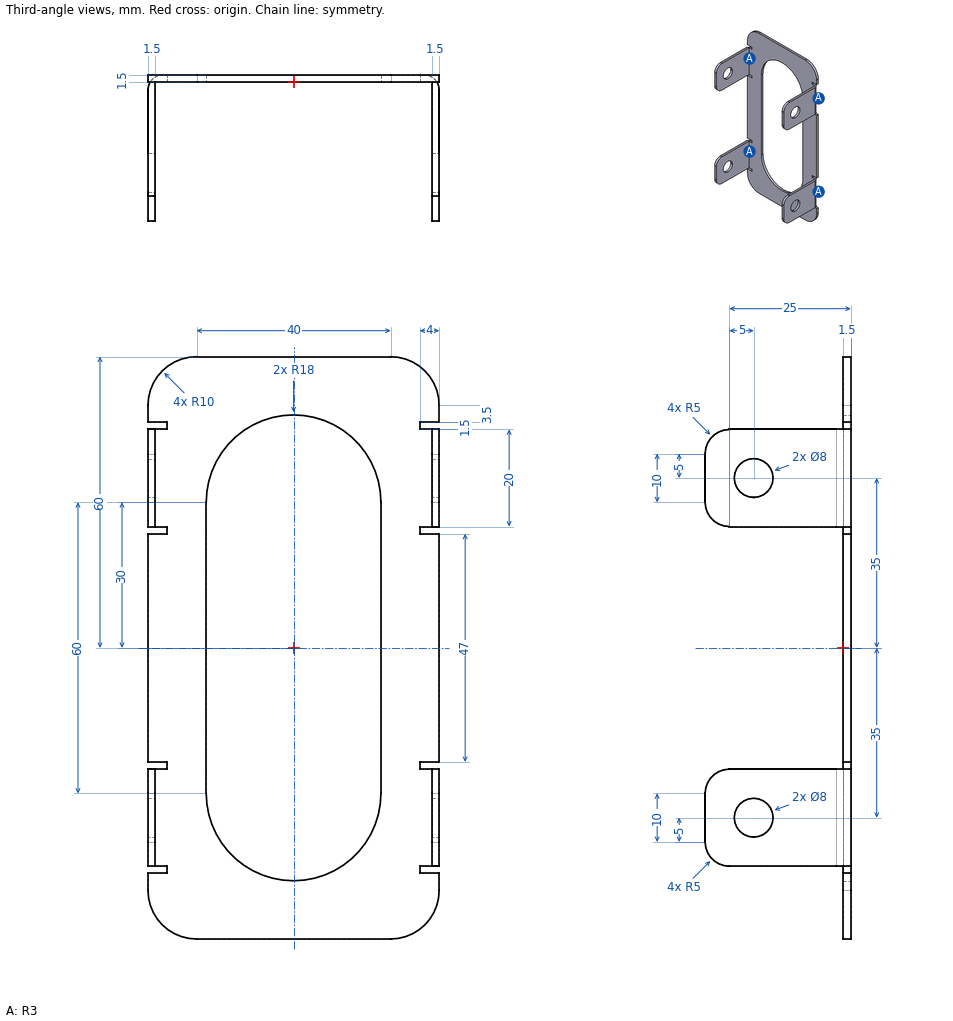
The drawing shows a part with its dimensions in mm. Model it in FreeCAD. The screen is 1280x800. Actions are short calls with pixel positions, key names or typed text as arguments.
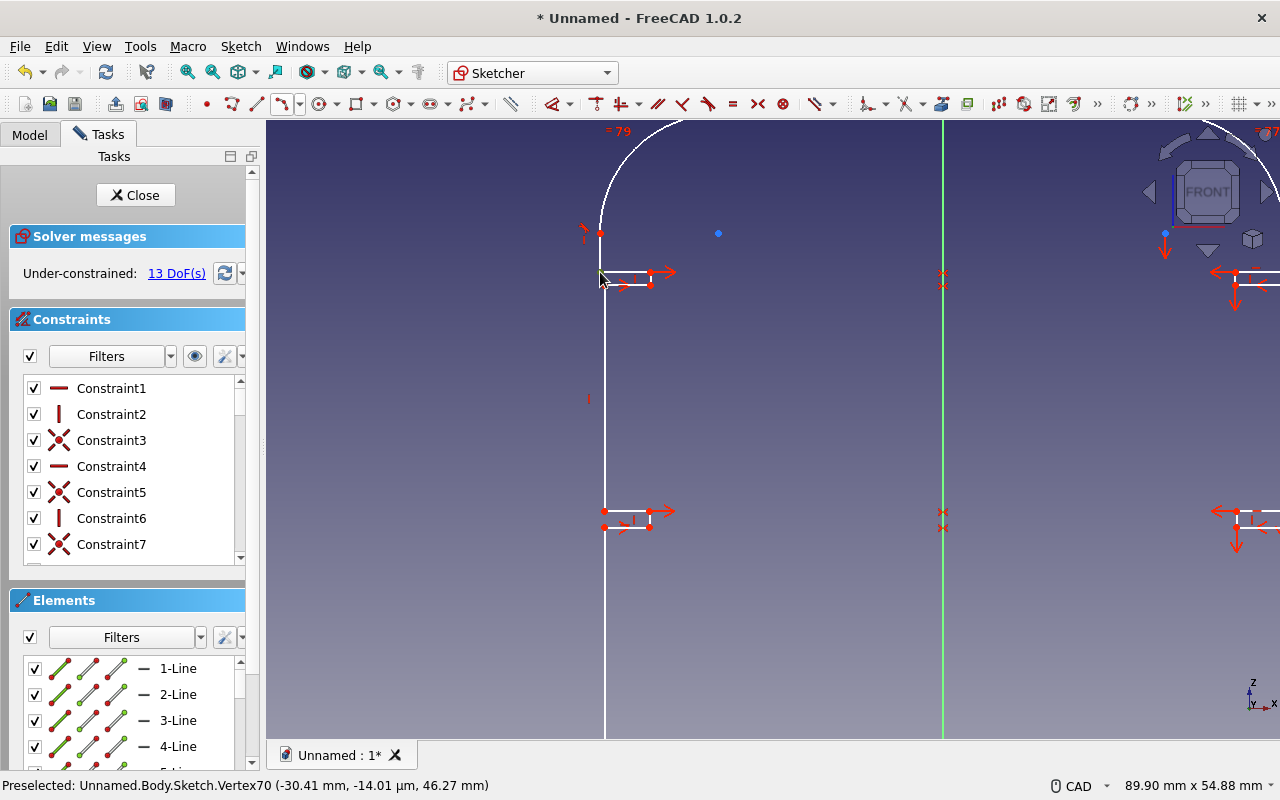
scroll(602, 272, down, 6)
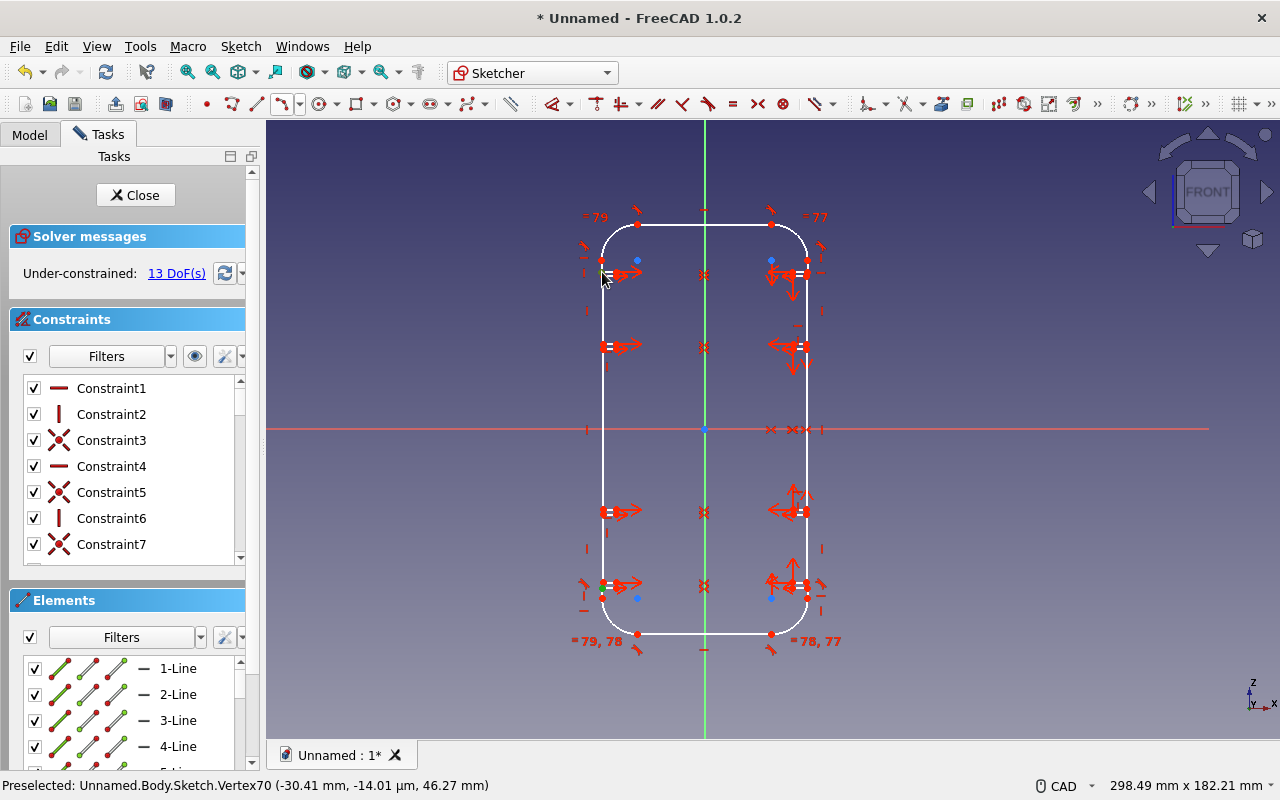
click(353, 429)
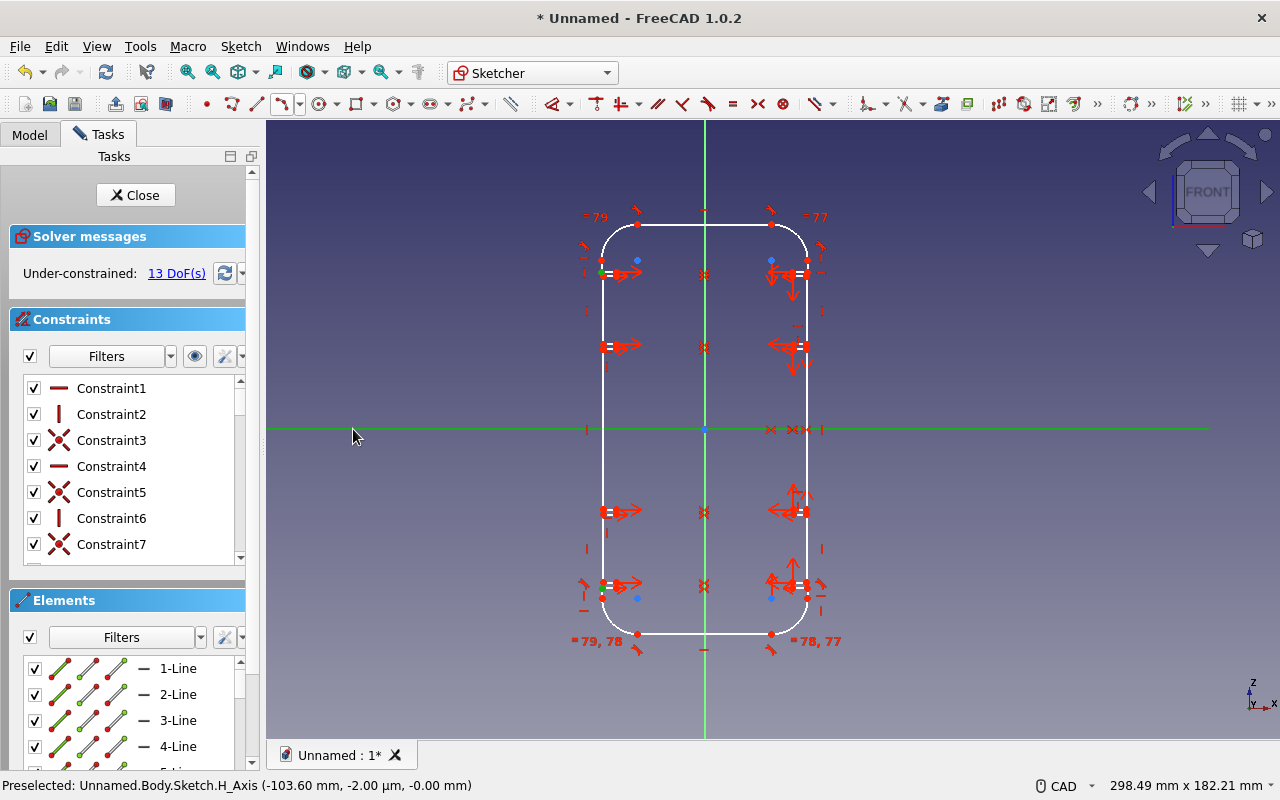
click(758, 104)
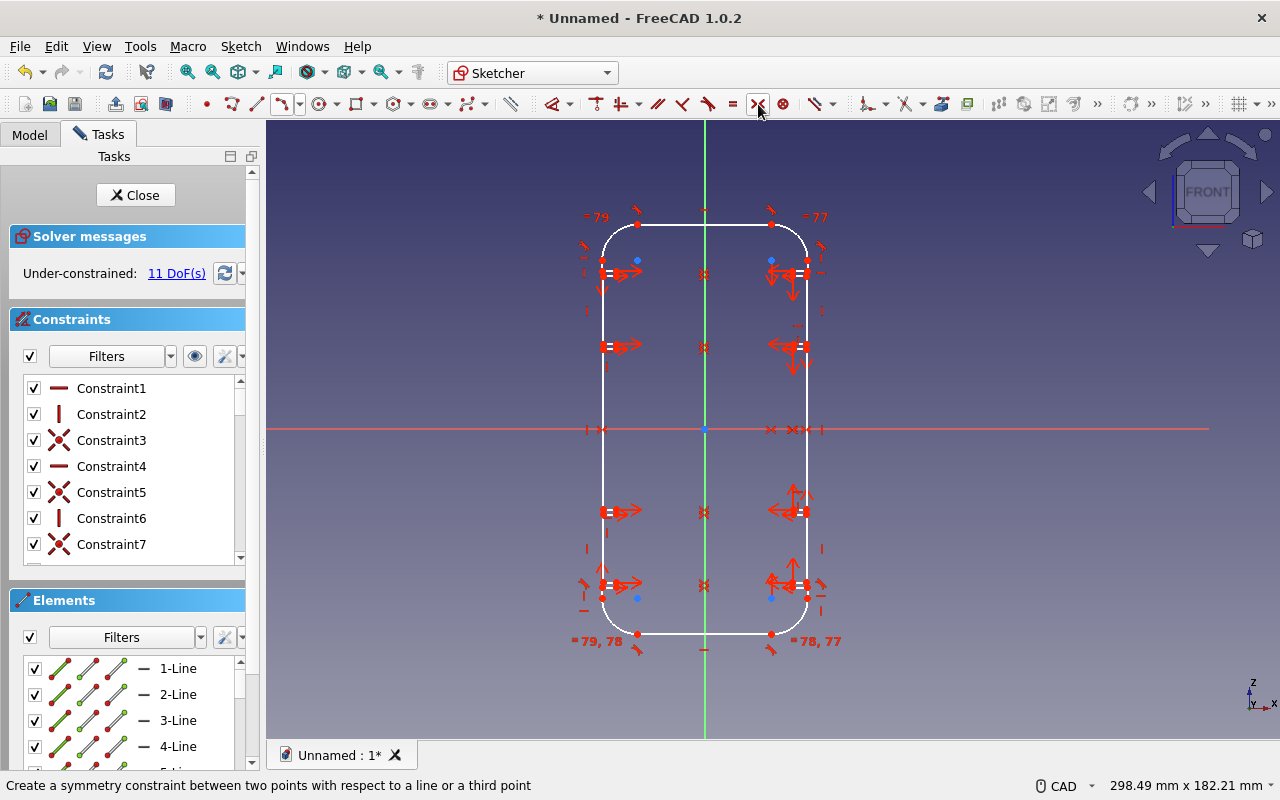
click(804, 244)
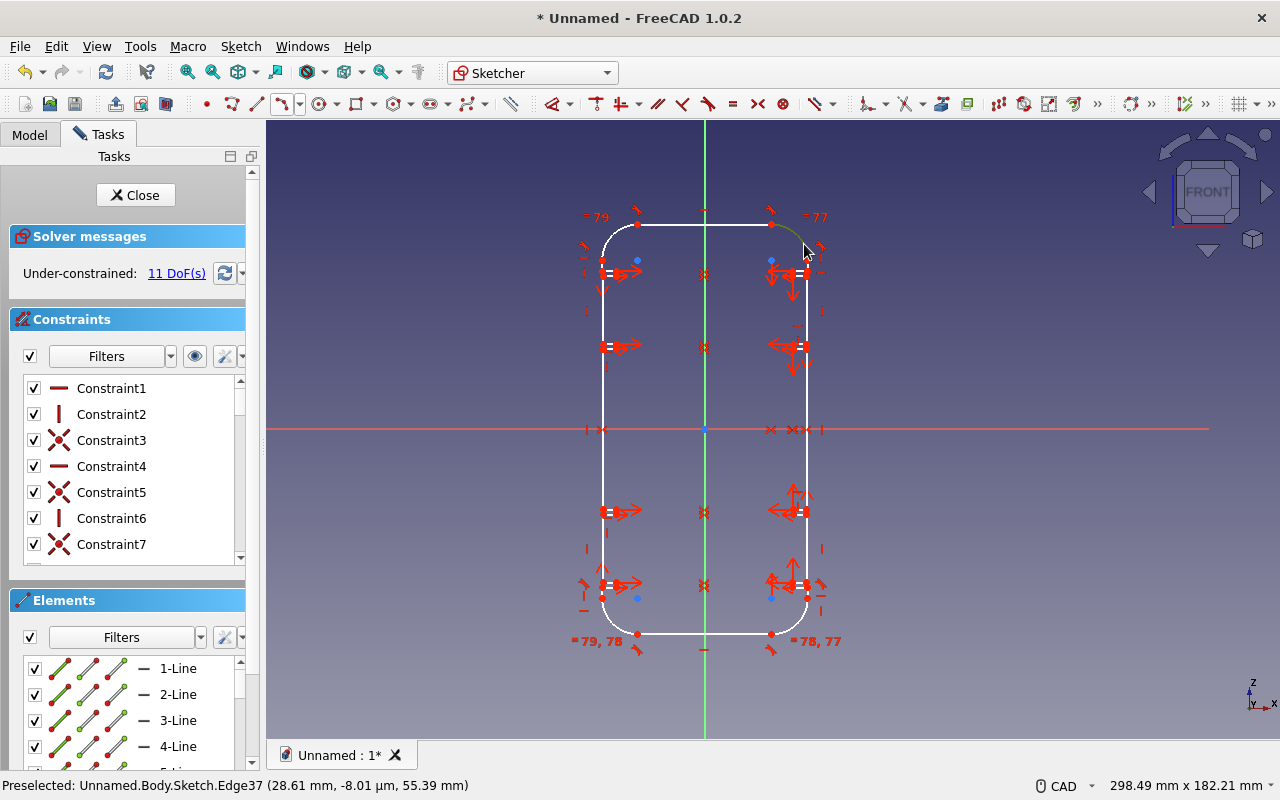
key(k)
key(r)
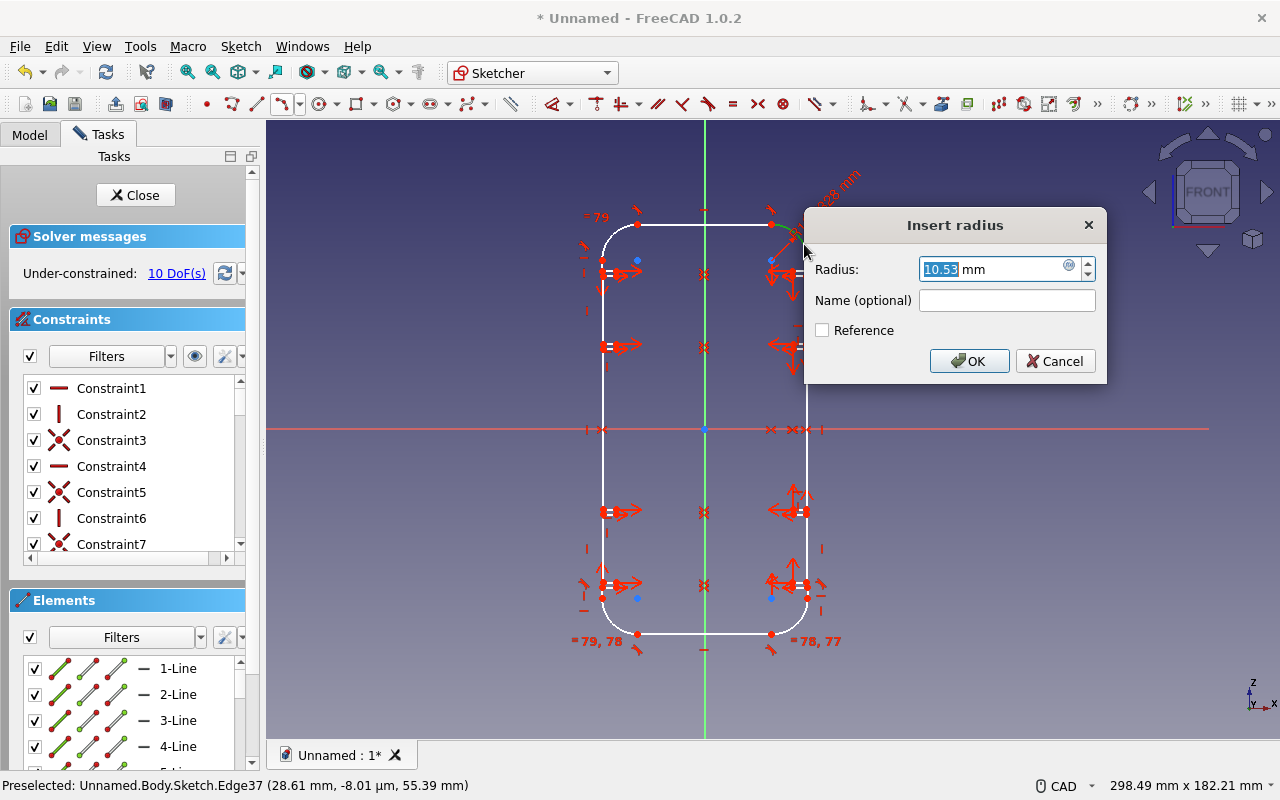
text(10)
key(Return)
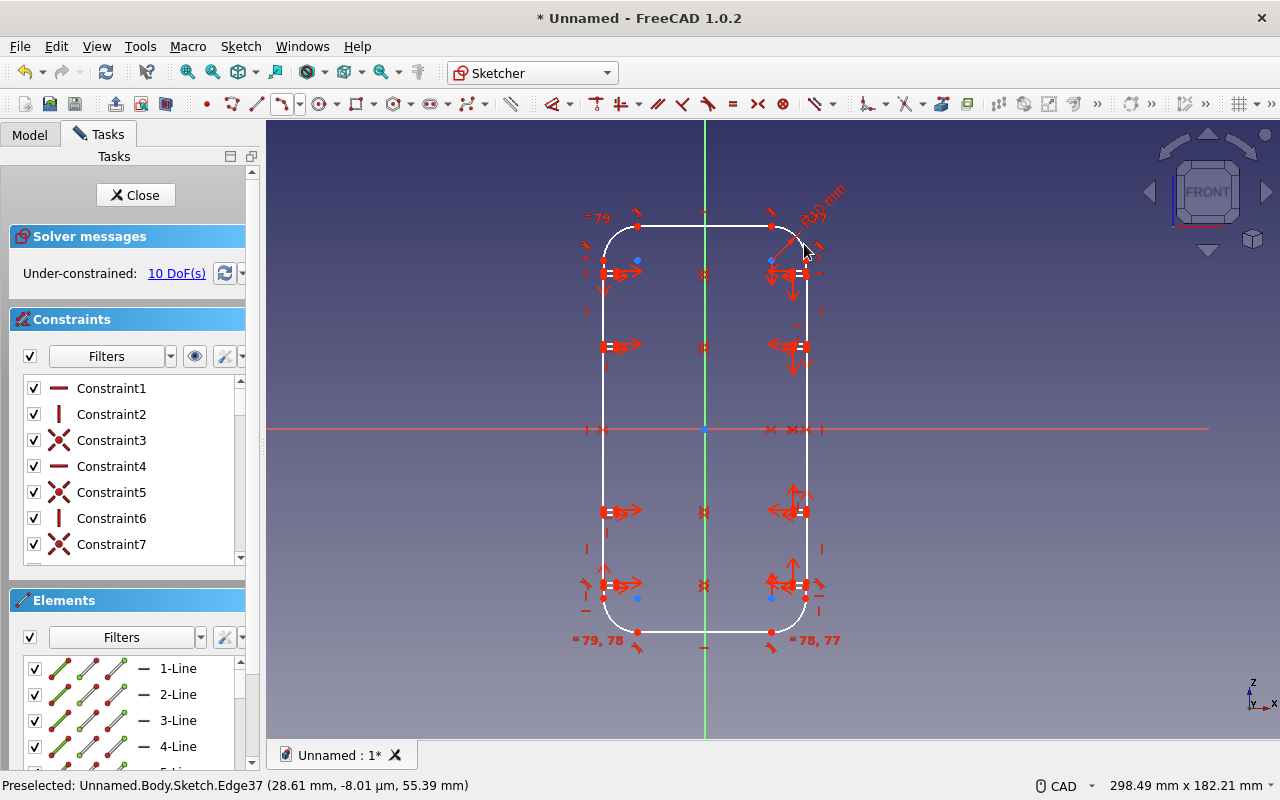
scroll(801, 271, up, 6)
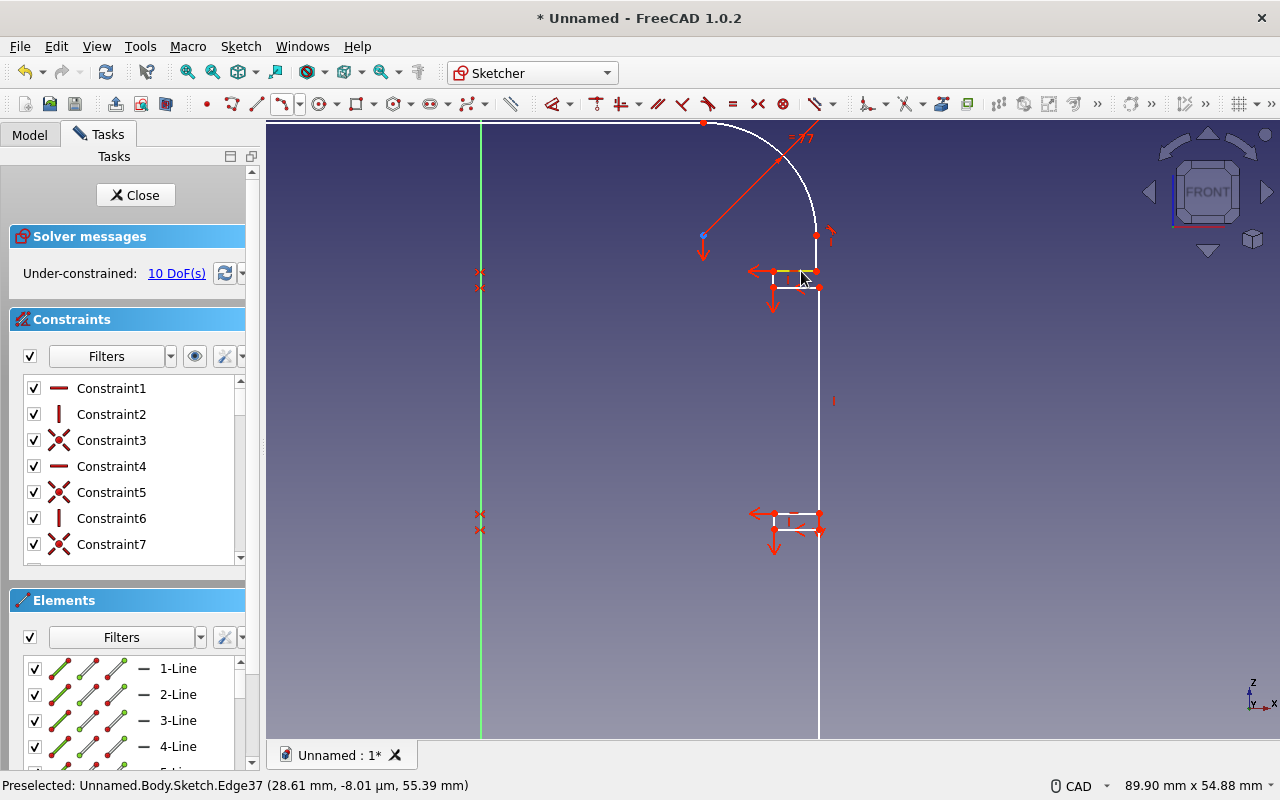
click(786, 271)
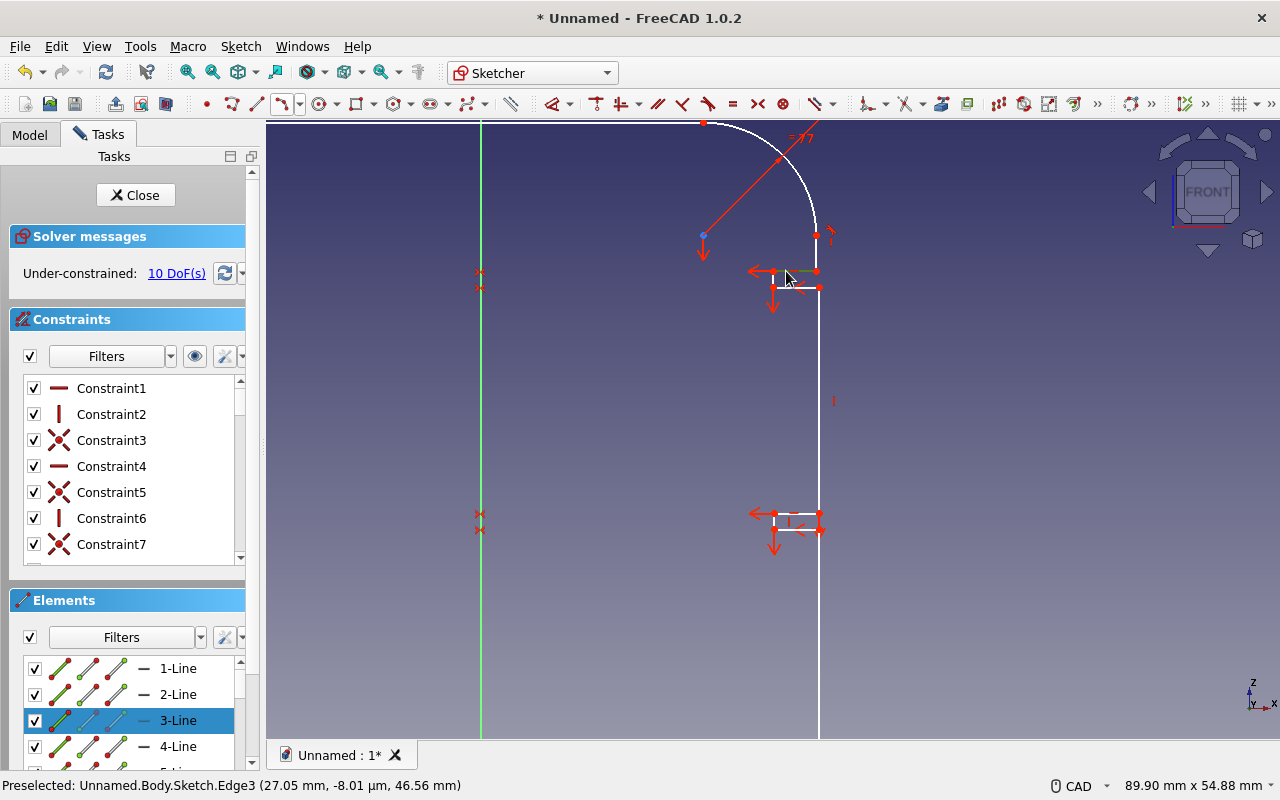
click(570, 104)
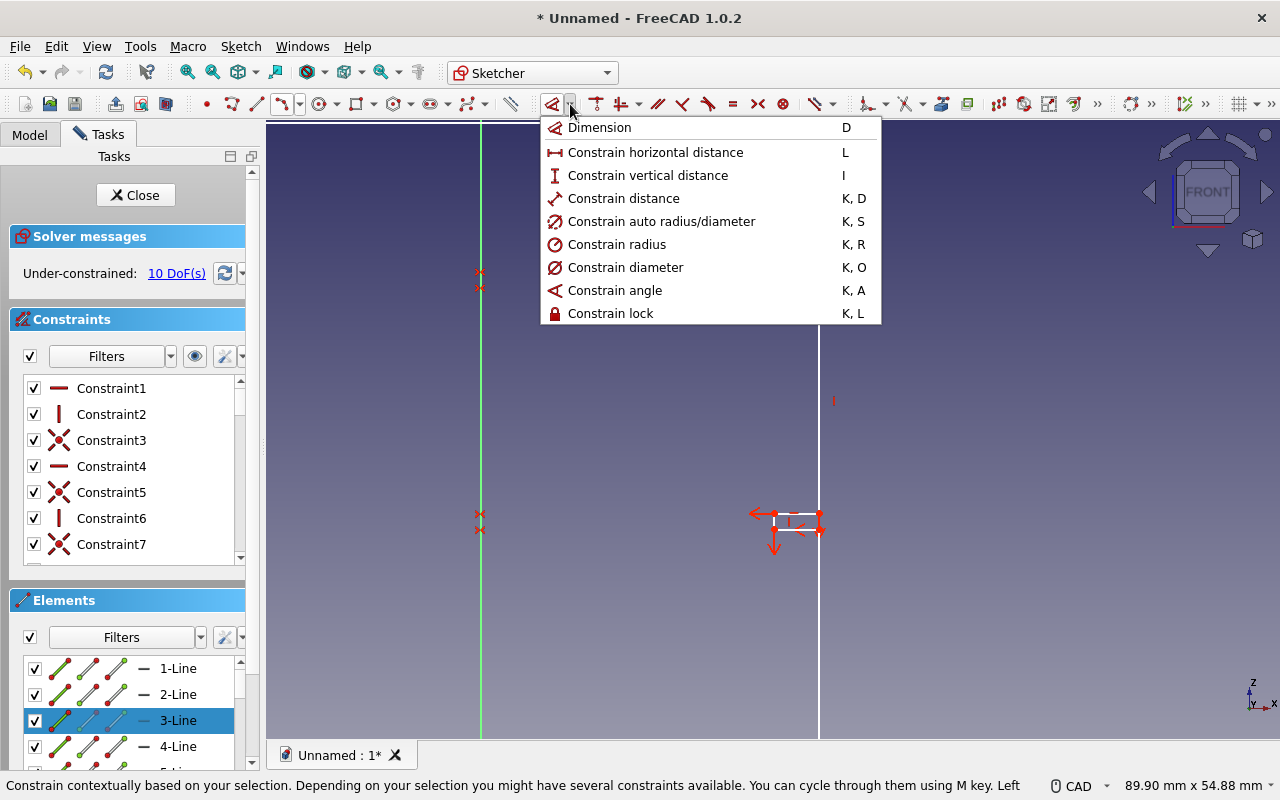
click(711, 152)